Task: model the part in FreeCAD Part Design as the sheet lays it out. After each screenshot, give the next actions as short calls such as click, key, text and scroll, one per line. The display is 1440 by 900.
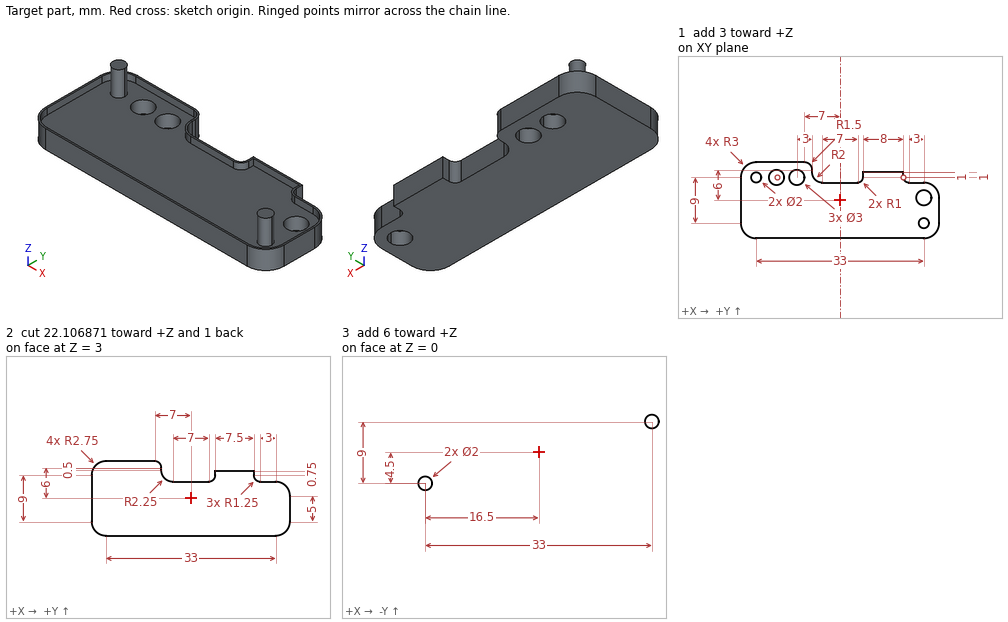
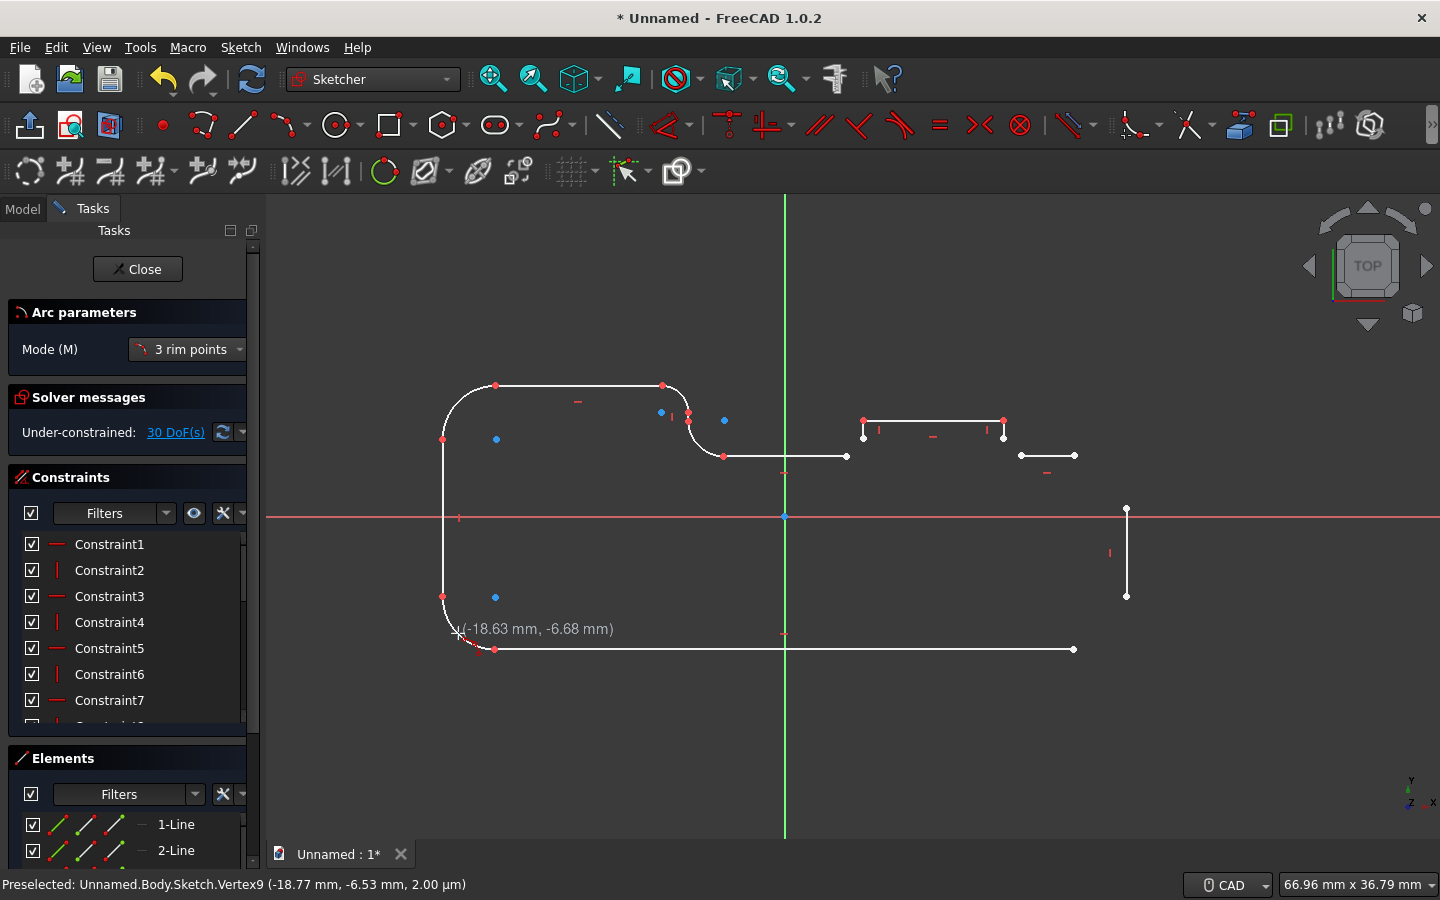
click(1074, 649)
click(1127, 596)
click(1111, 633)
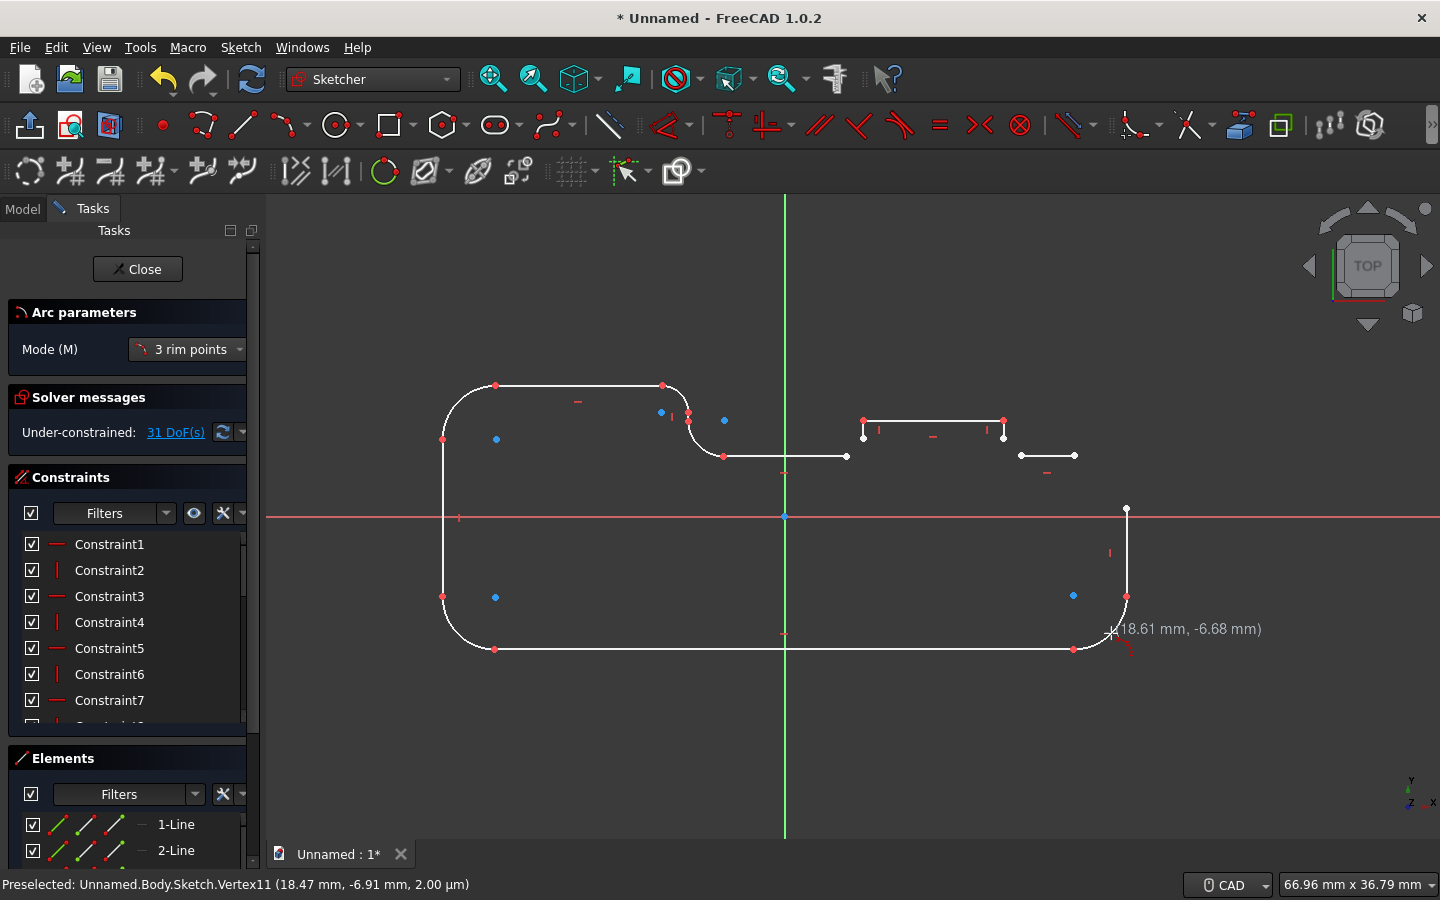
scroll(1127, 508, up, 3)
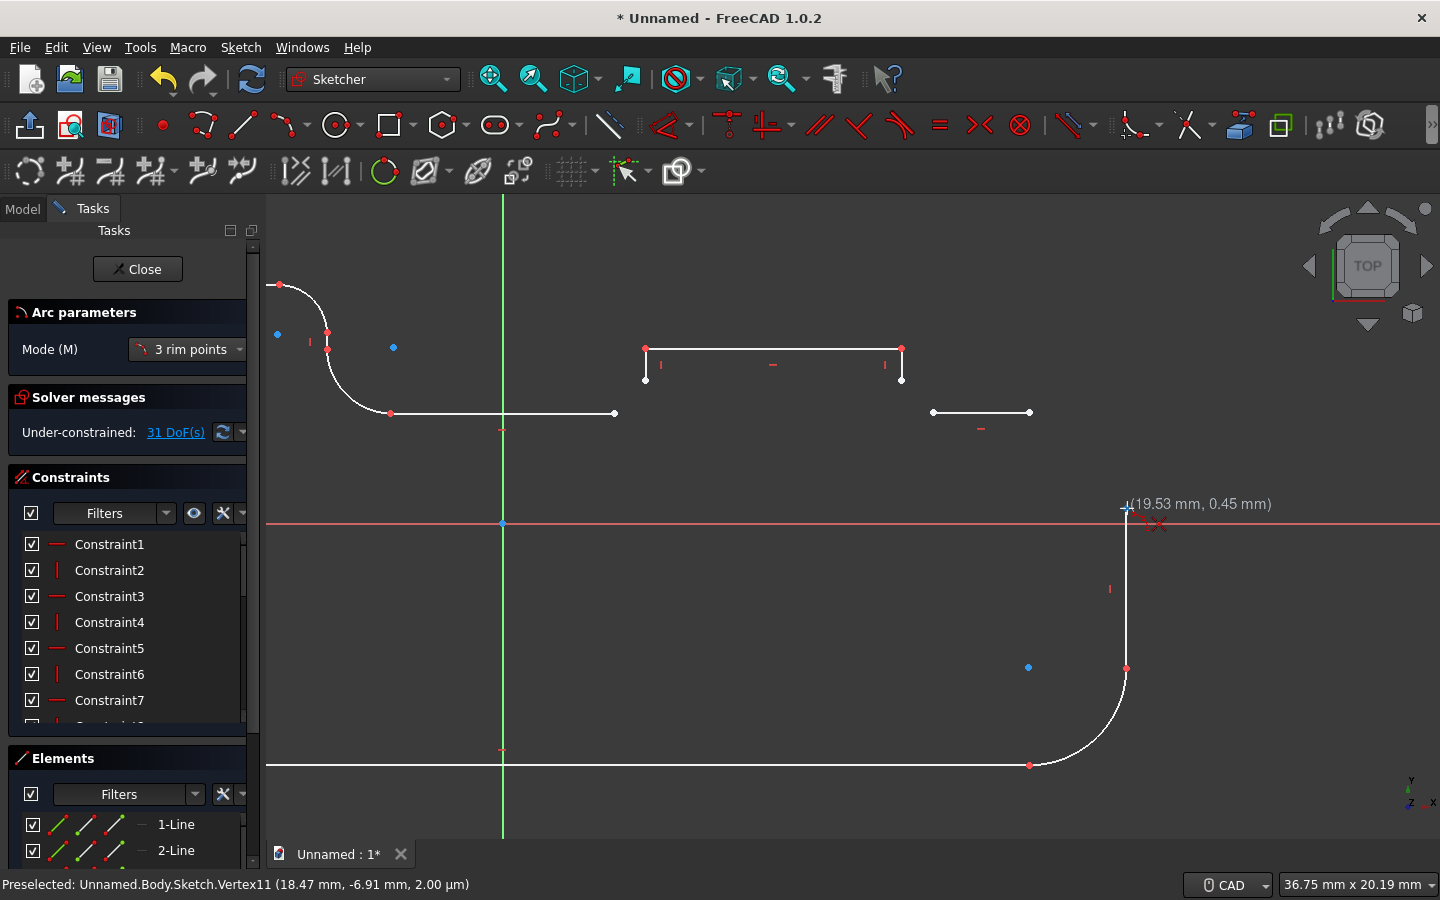
click(1126, 509)
click(1030, 413)
click(1097, 440)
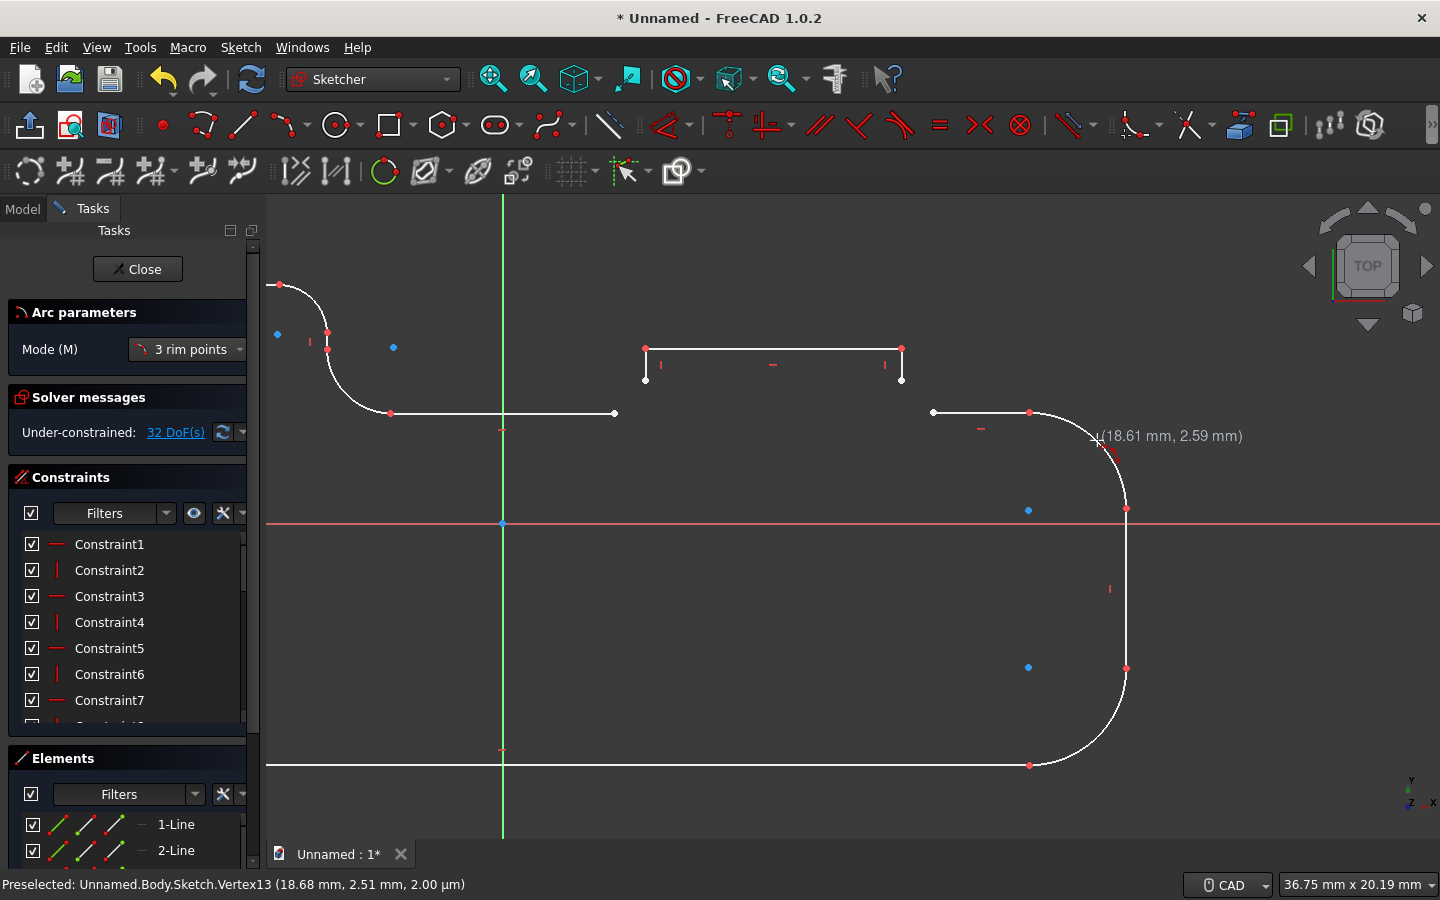
click(934, 413)
click(902, 381)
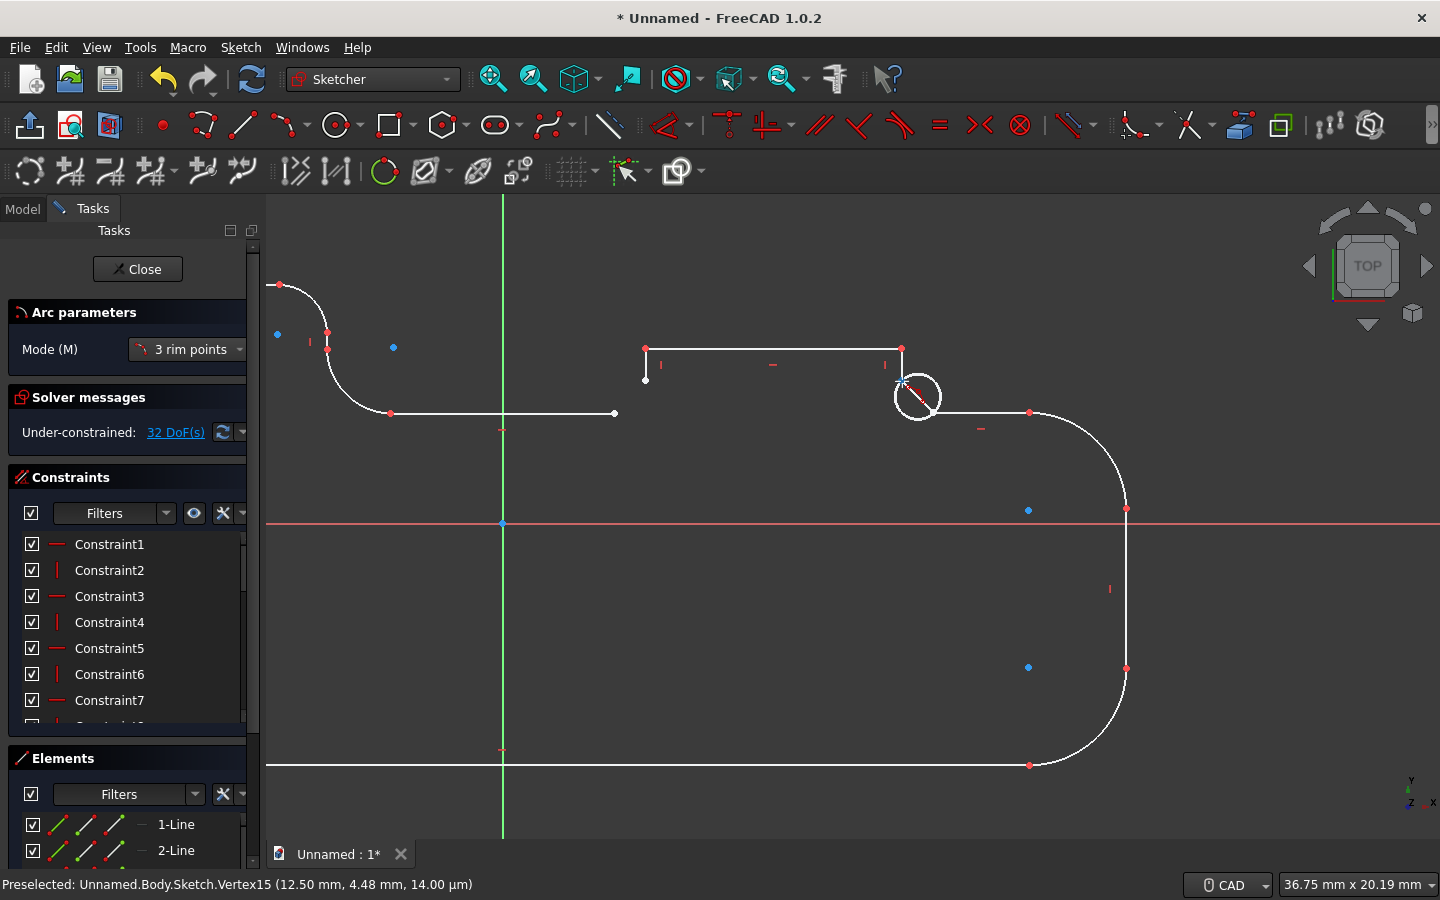
scroll(911, 403, up, 3)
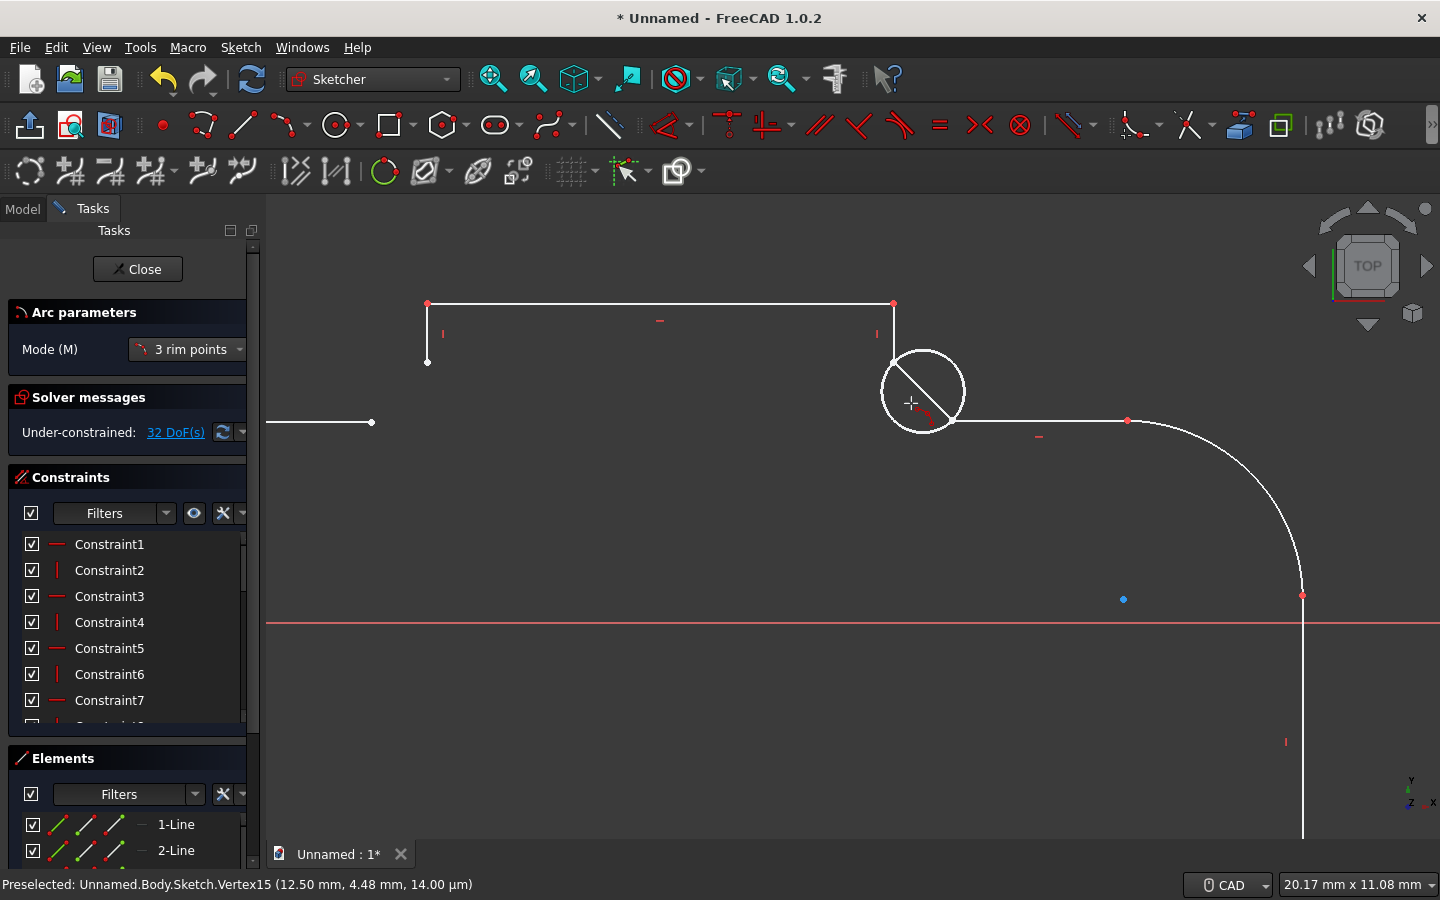
click(911, 402)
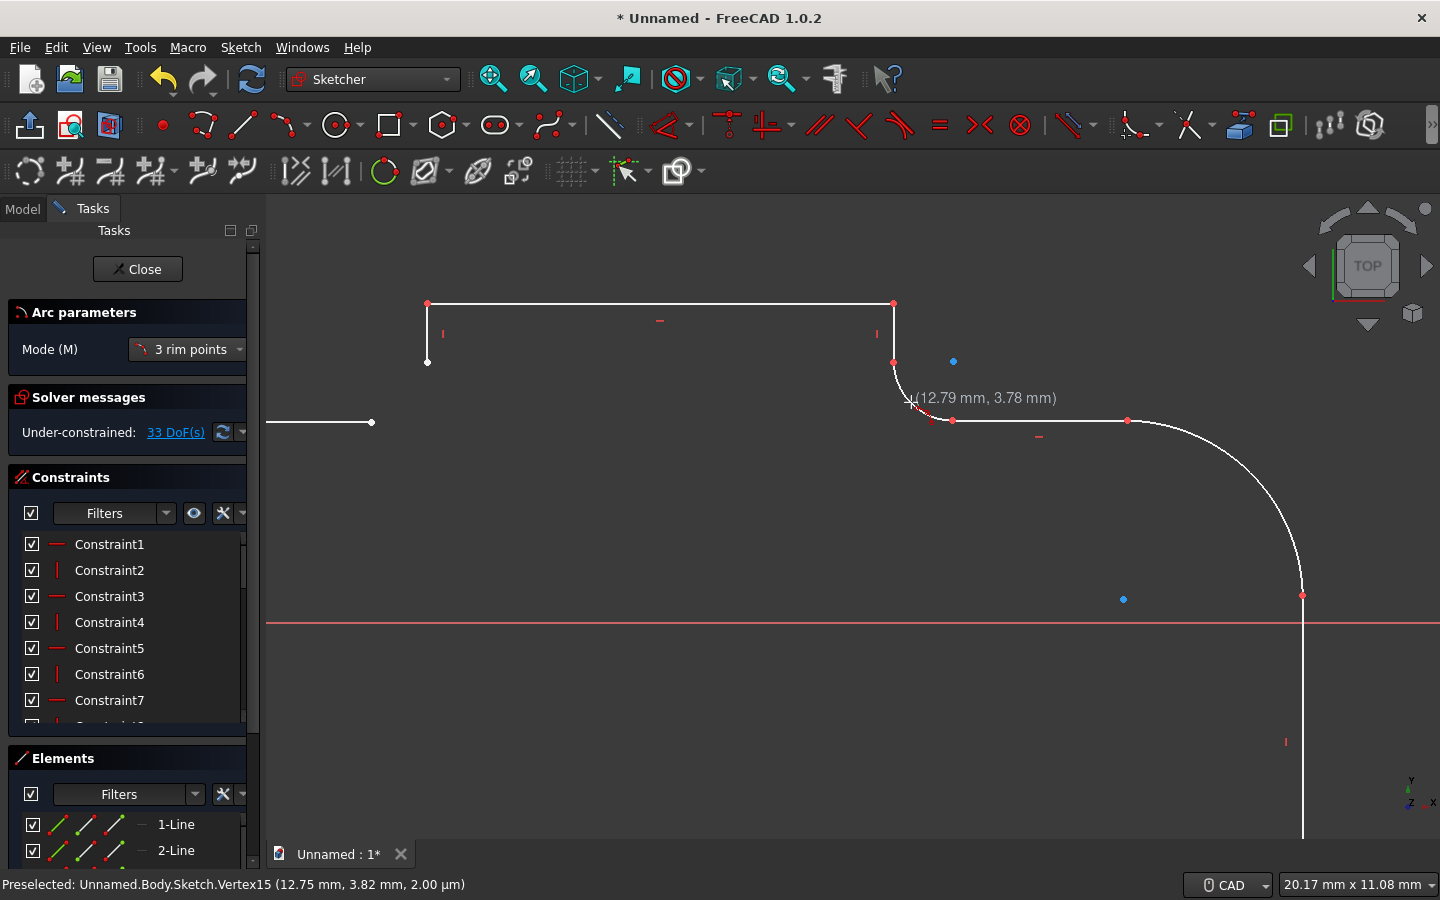
click(427, 362)
click(371, 422)
click(411, 402)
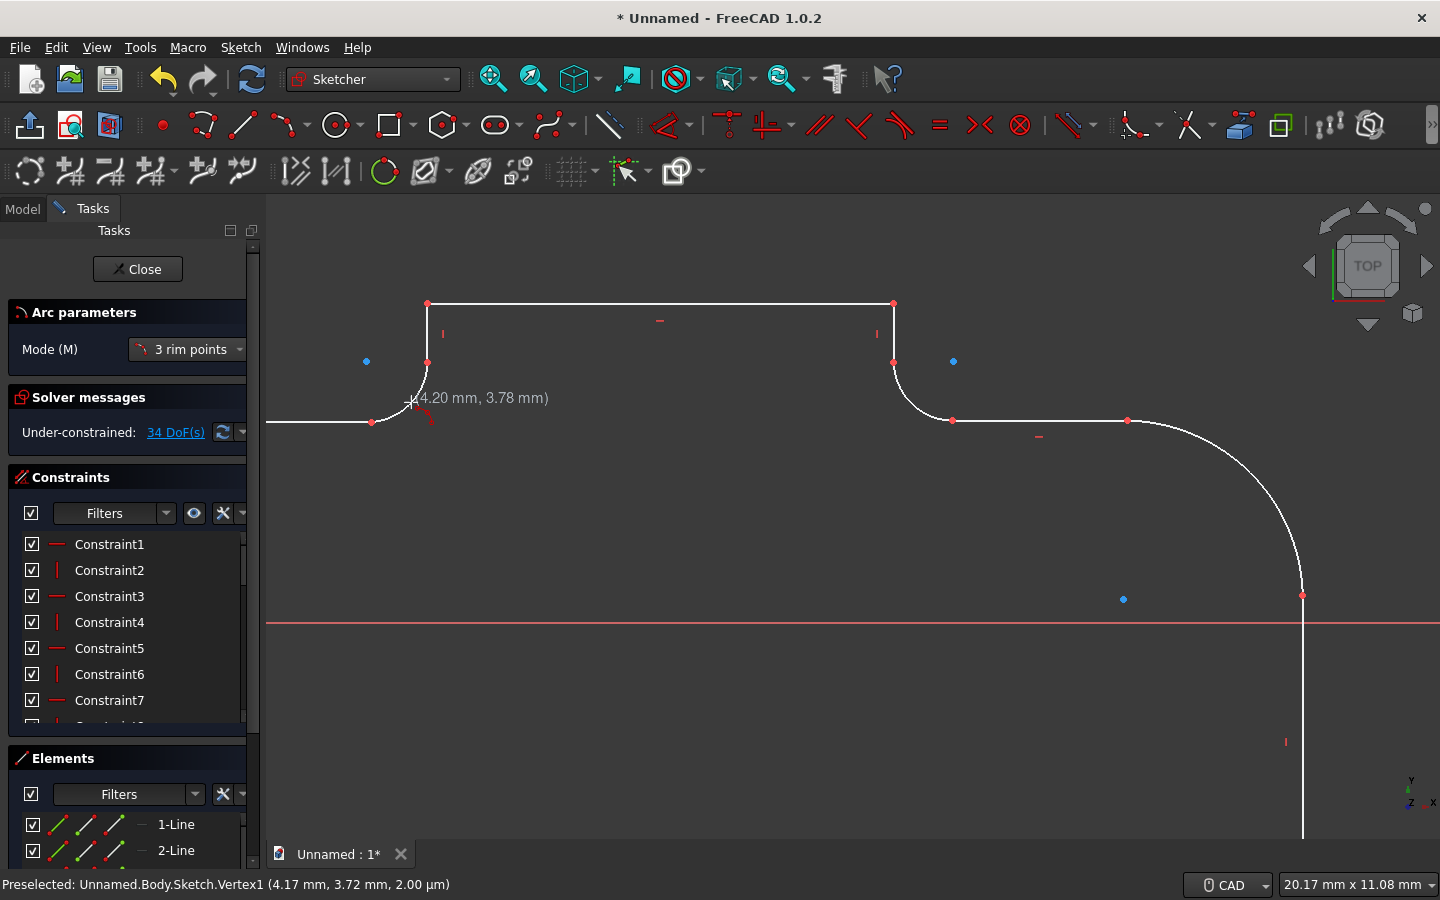
click(336, 126)